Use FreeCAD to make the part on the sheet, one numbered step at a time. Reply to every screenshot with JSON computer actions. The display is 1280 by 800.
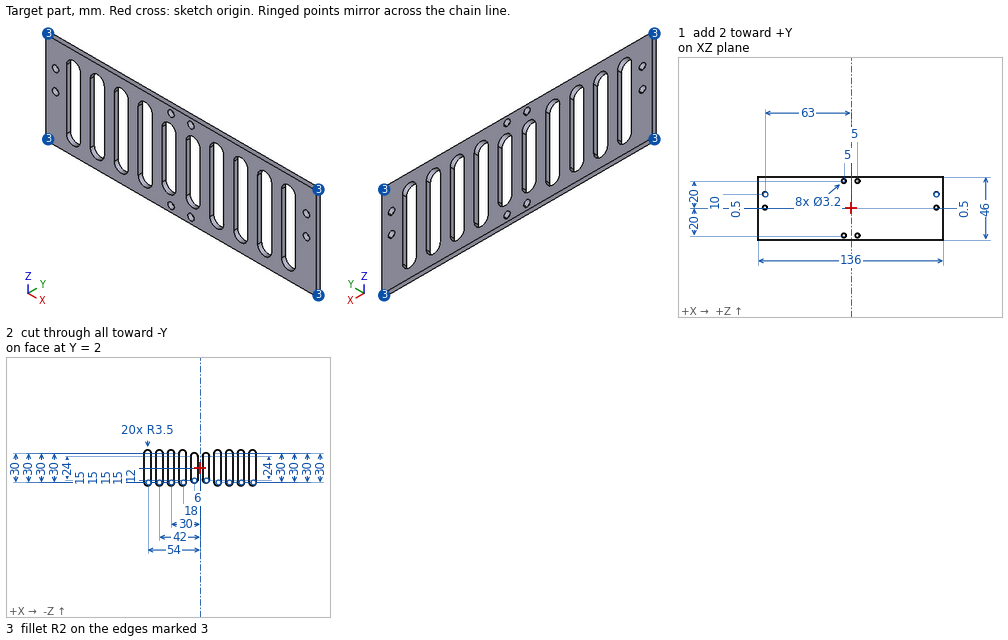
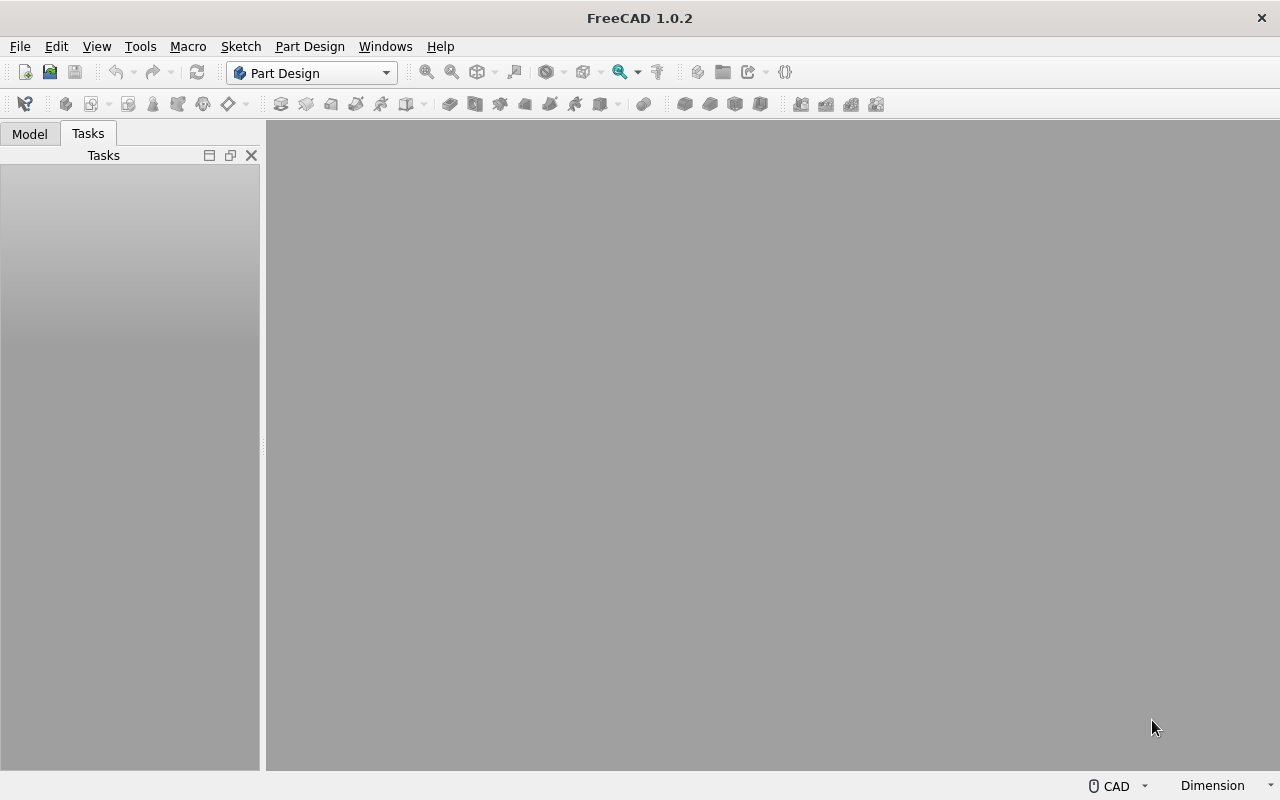
{"action": "left_click", "coordinate": [25, 72]}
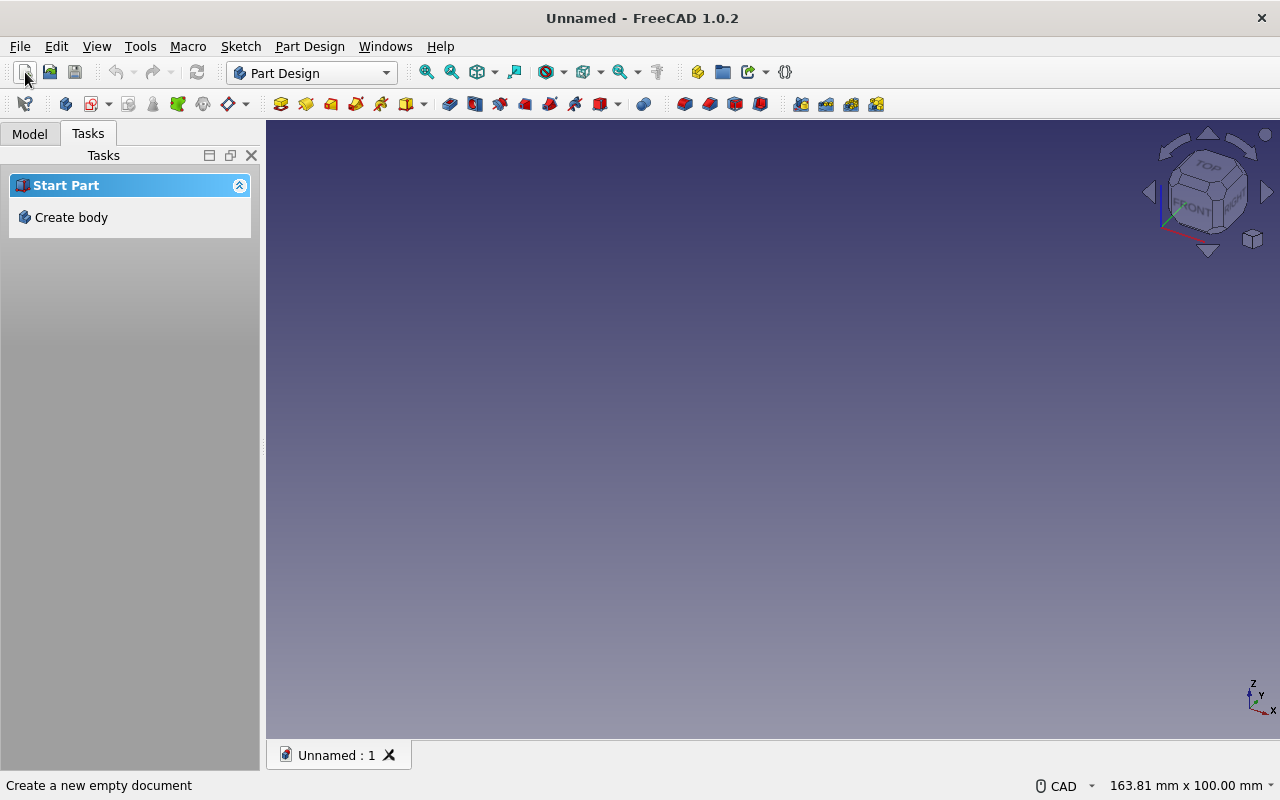
{"action": "left_click", "coordinate": [90, 104]}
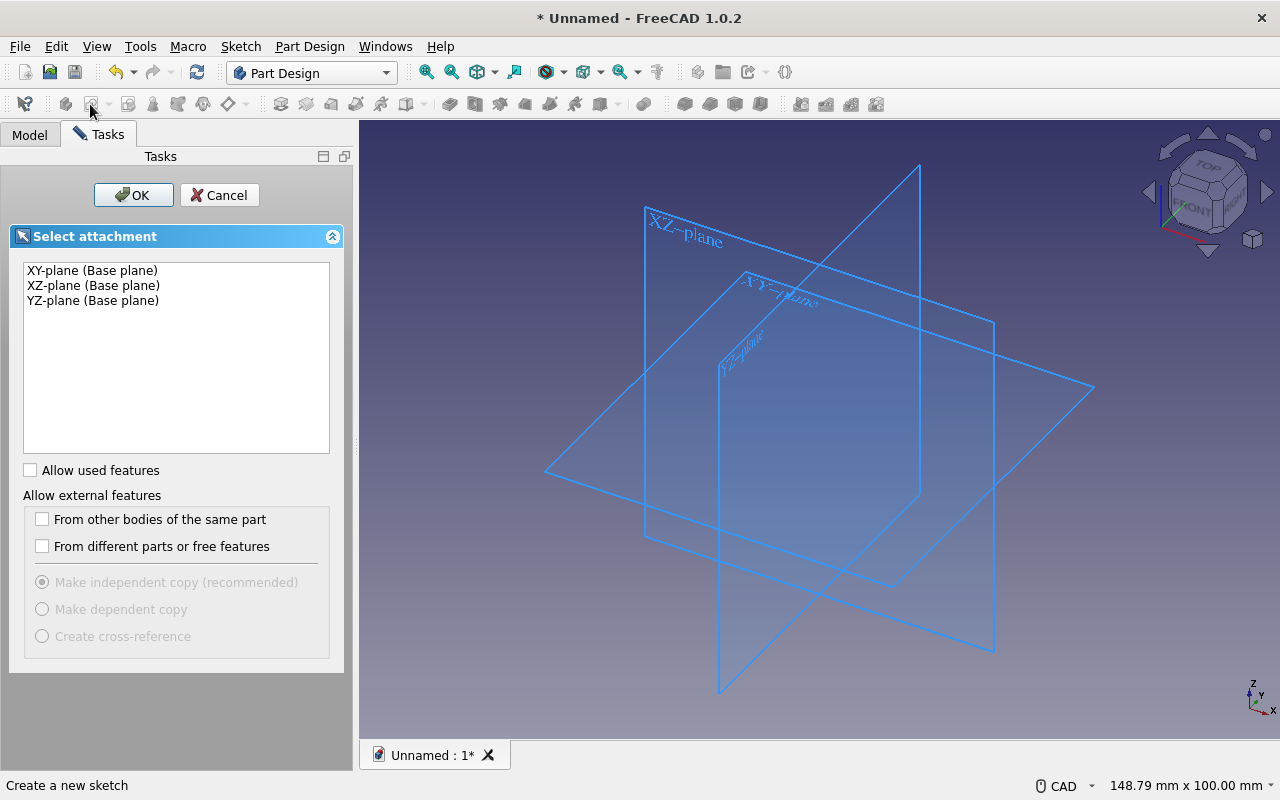
{"action": "left_click", "coordinate": [84, 286]}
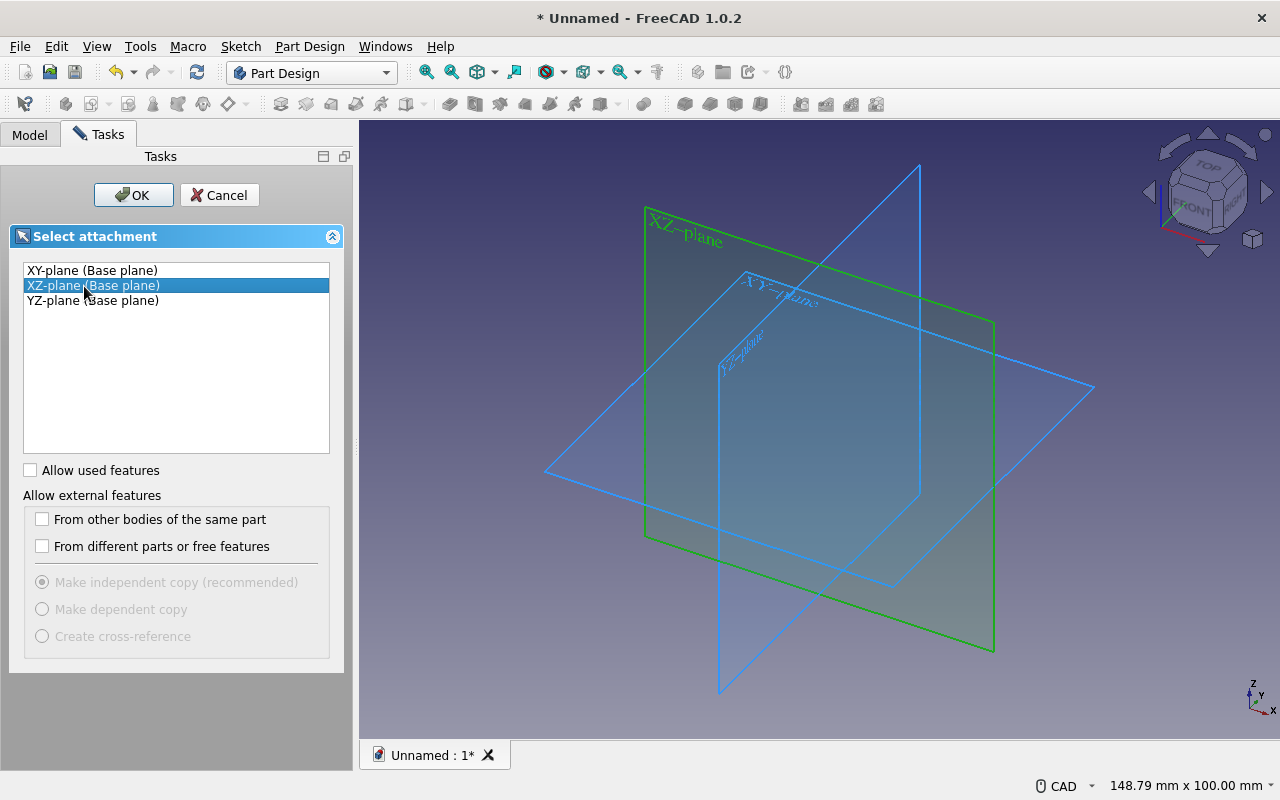
{"action": "left_click", "coordinate": [134, 195]}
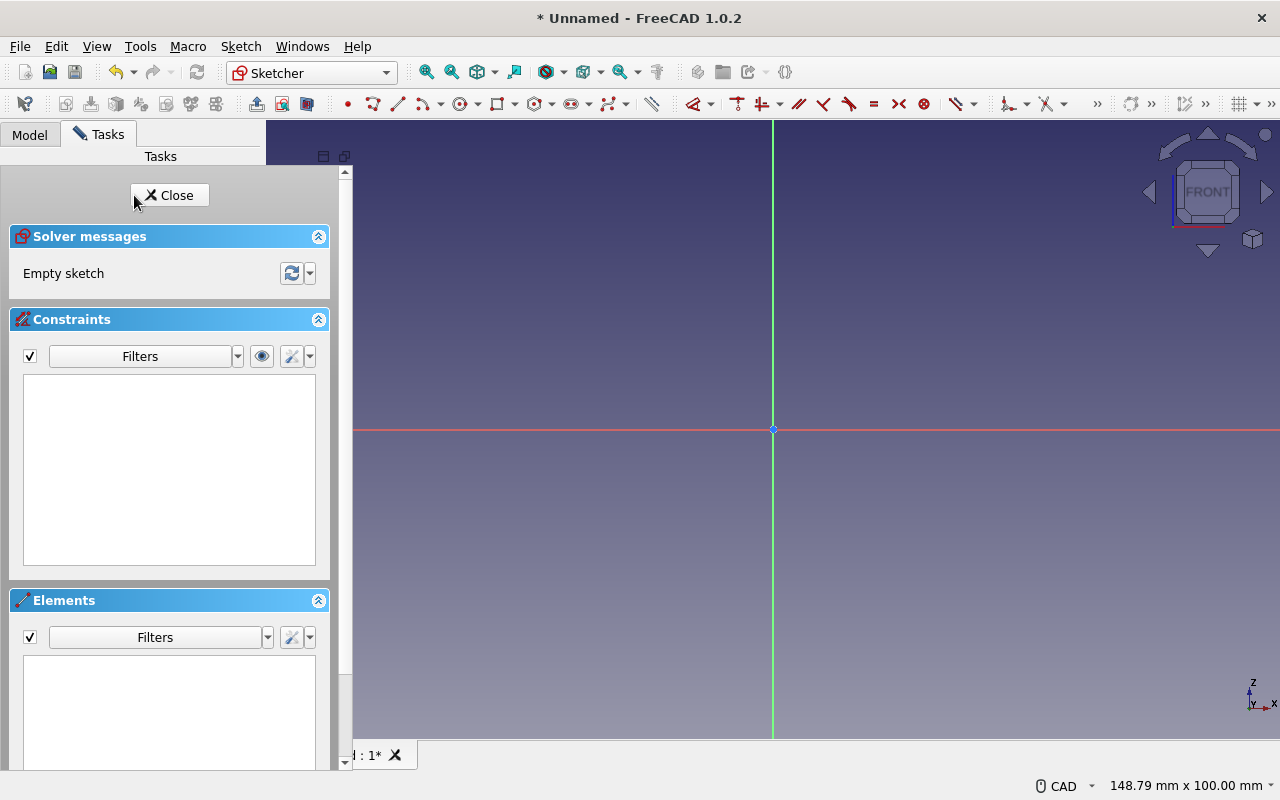
{"action": "scroll", "coordinate": [565, 429], "scroll_direction": "down", "scroll_amount": 2}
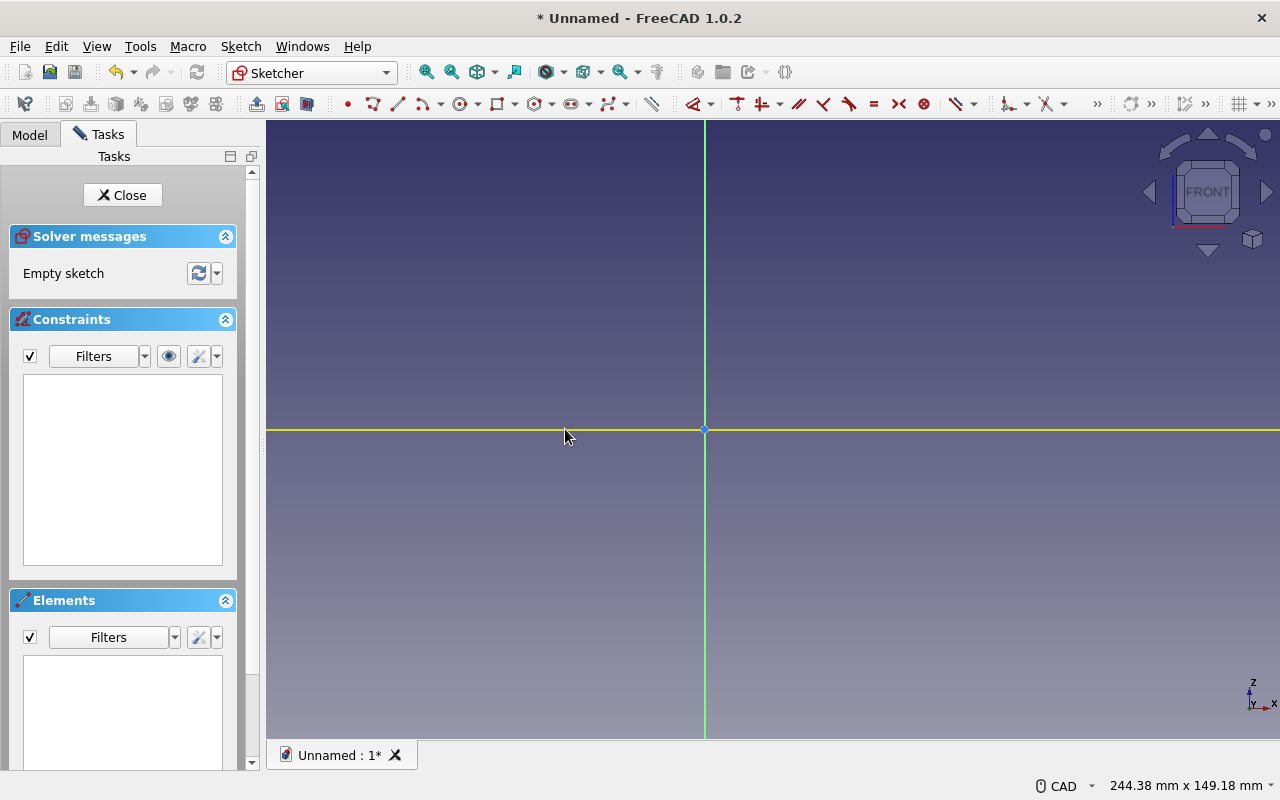
{"action": "key", "text": "g v"}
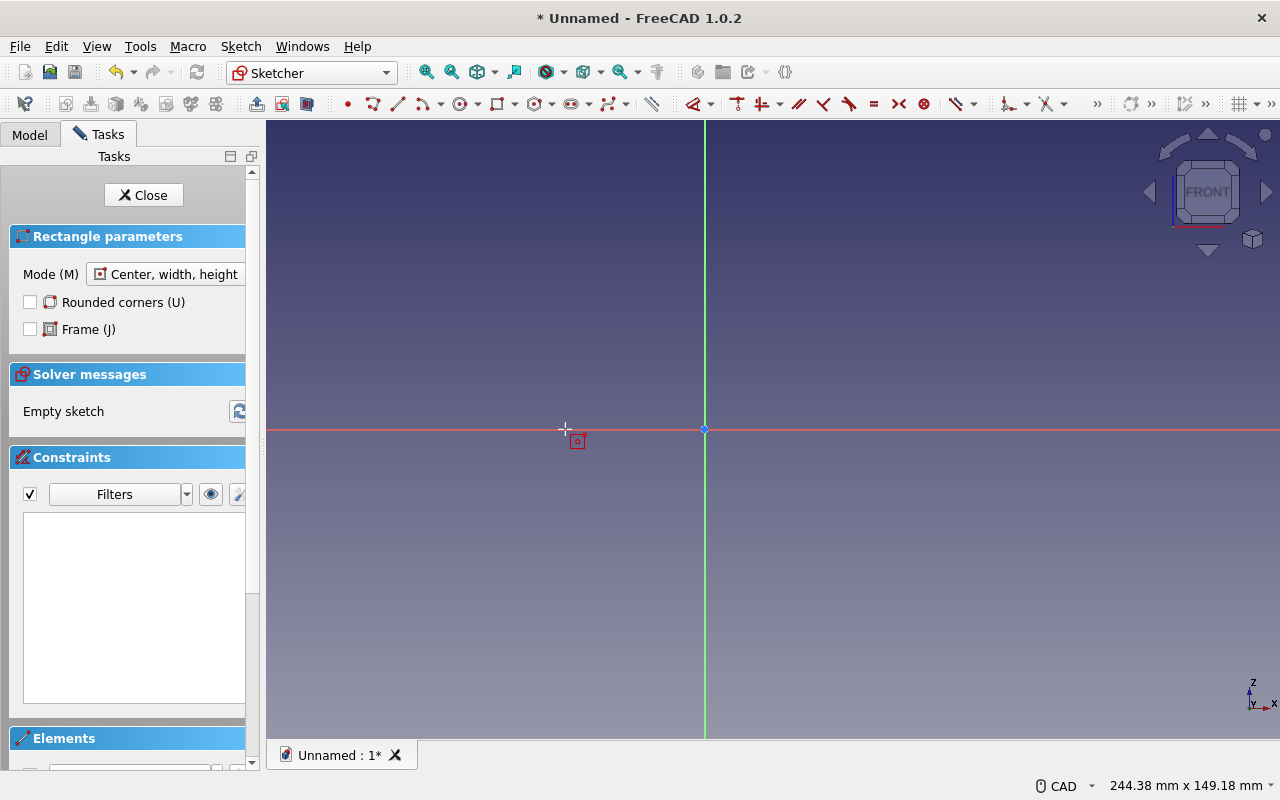
{"action": "left_click", "coordinate": [705, 430]}
{"action": "mouse_move", "coordinate": [987, 334]}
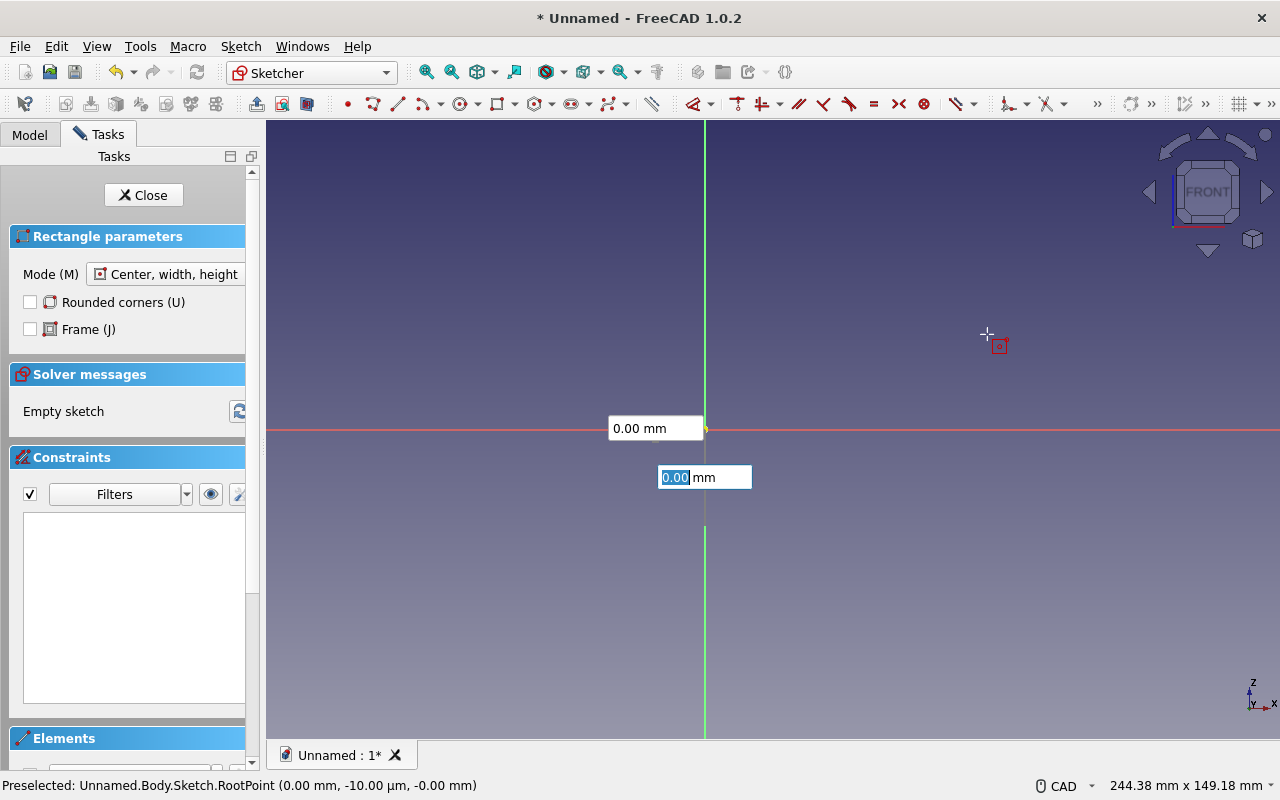
{"action": "type", "text": "136"}
{"action": "key", "text": "Tab"}
{"action": "type", "text": "46"}
{"action": "key", "text": "Return"}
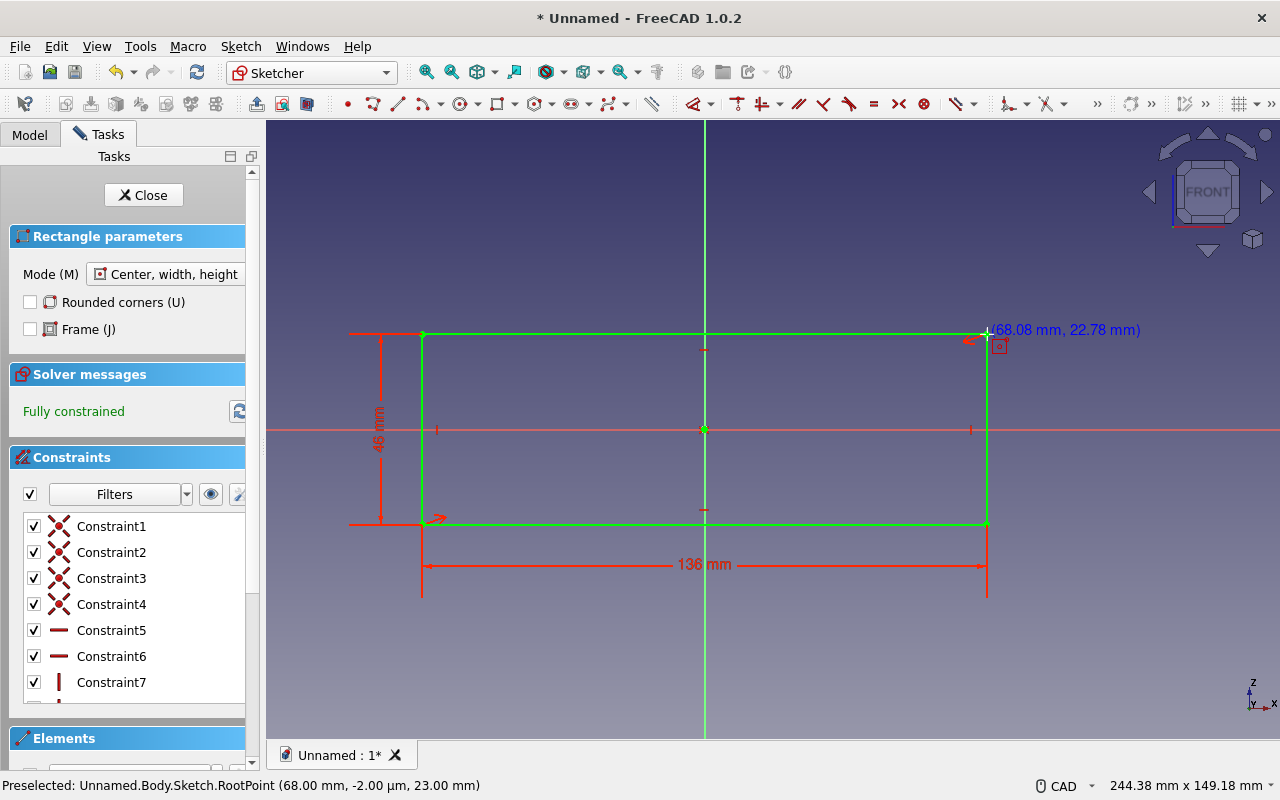
{"action": "left_click", "coordinate": [460, 104]}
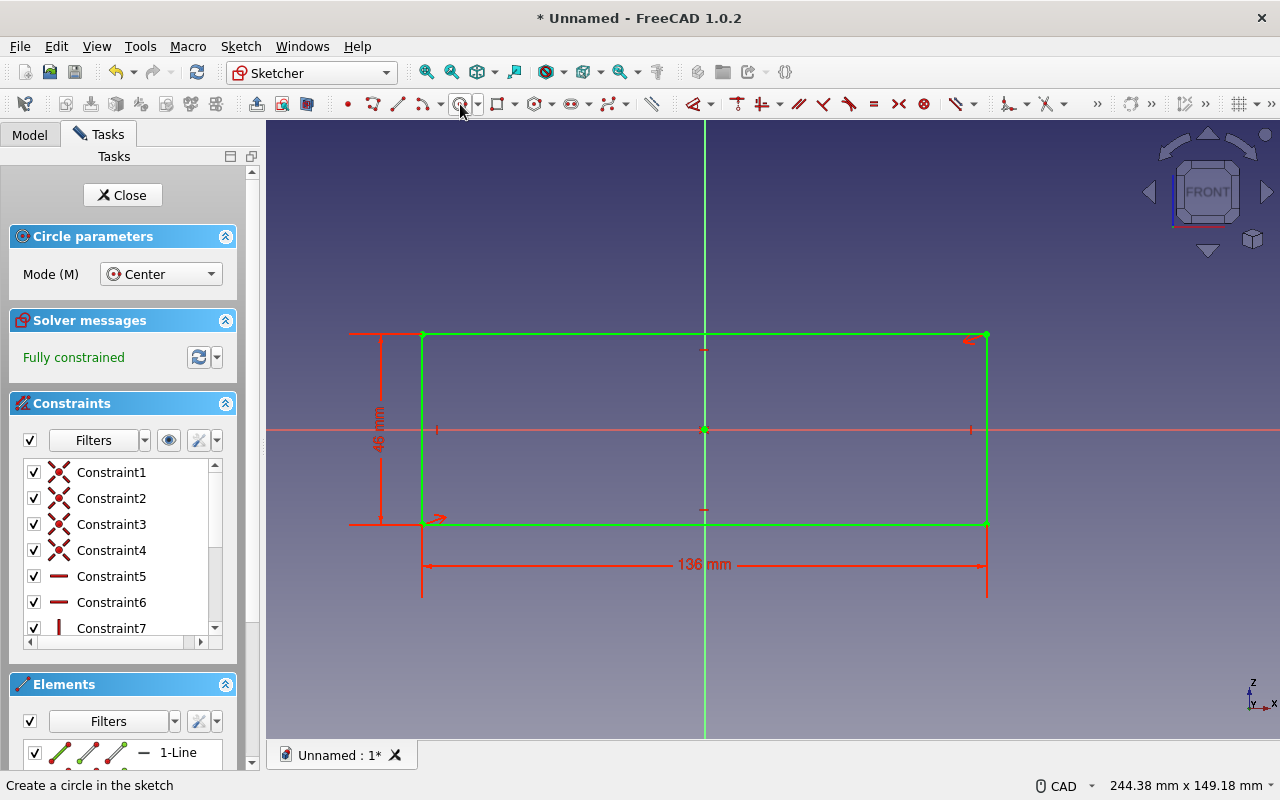
{"action": "scroll", "coordinate": [684, 347], "scroll_direction": "up", "scroll_amount": 7}